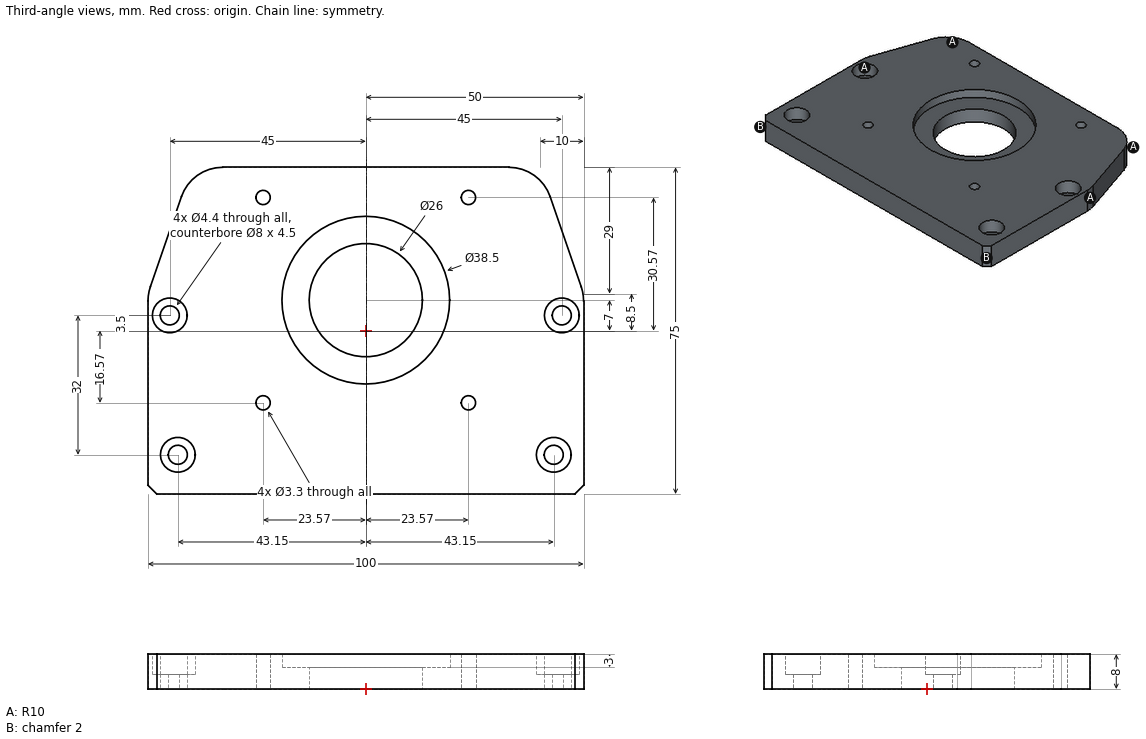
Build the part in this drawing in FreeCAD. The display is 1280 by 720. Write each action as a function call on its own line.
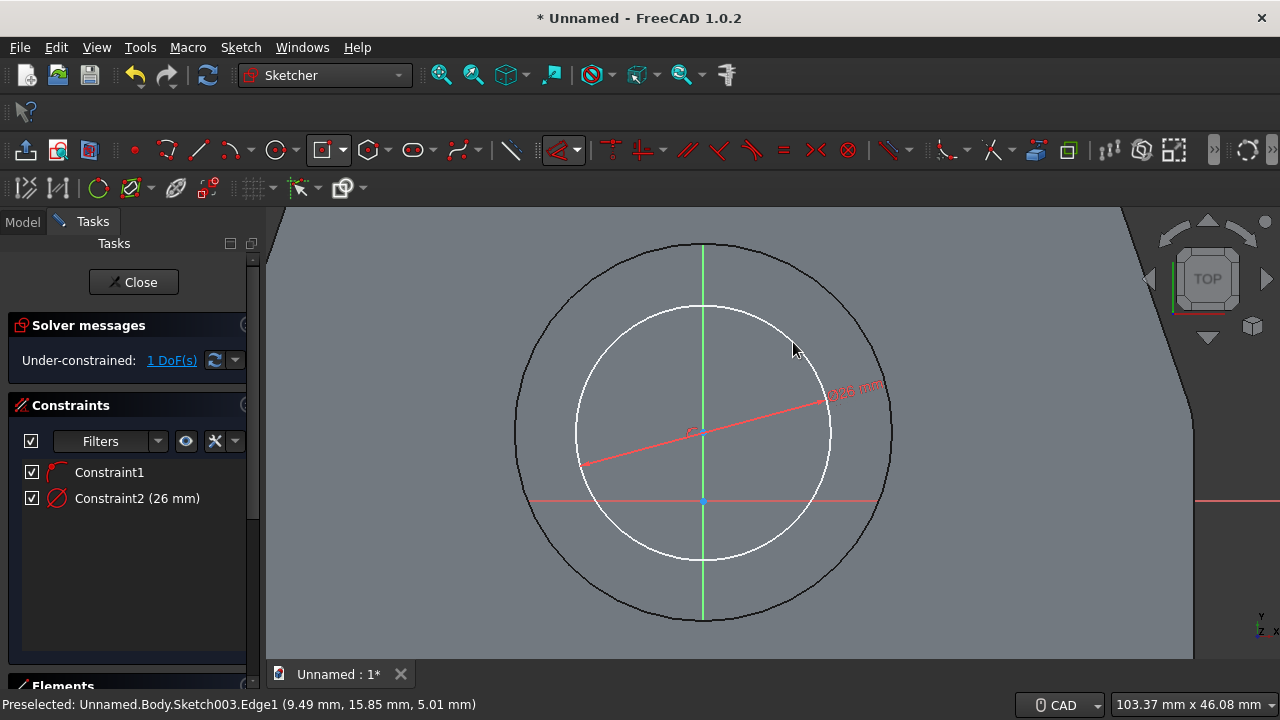
click(703, 433)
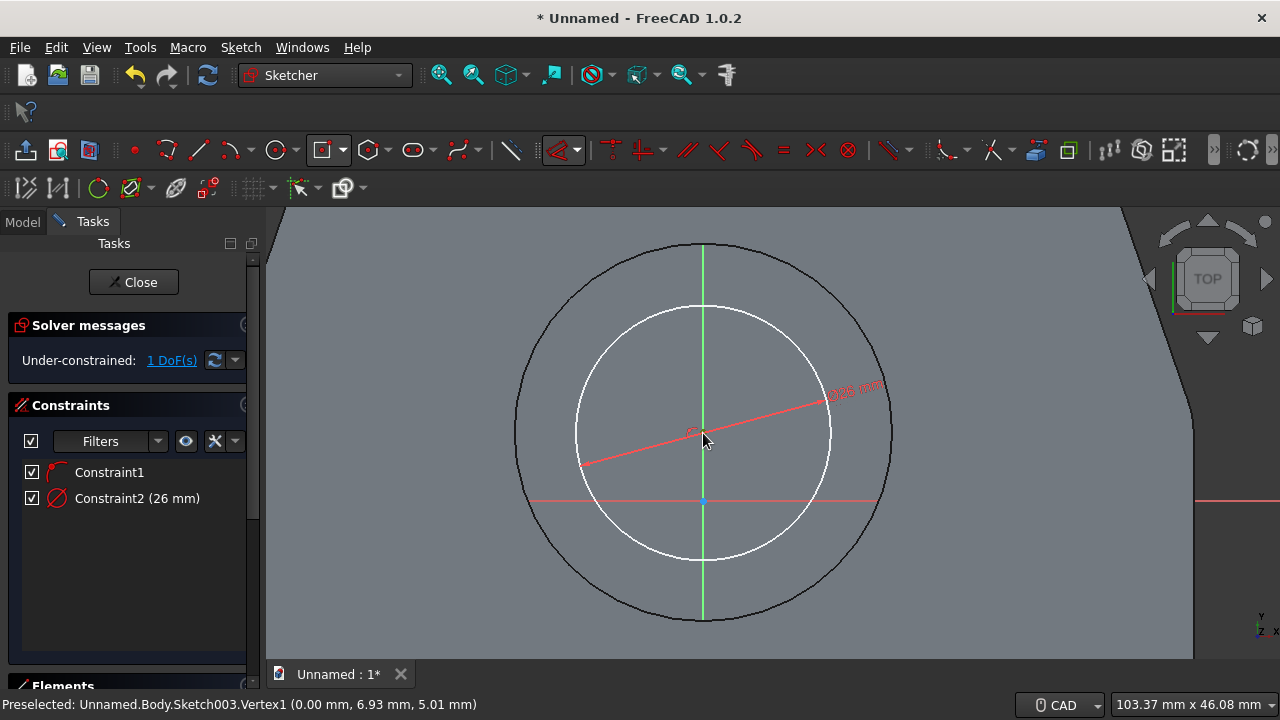
key(i)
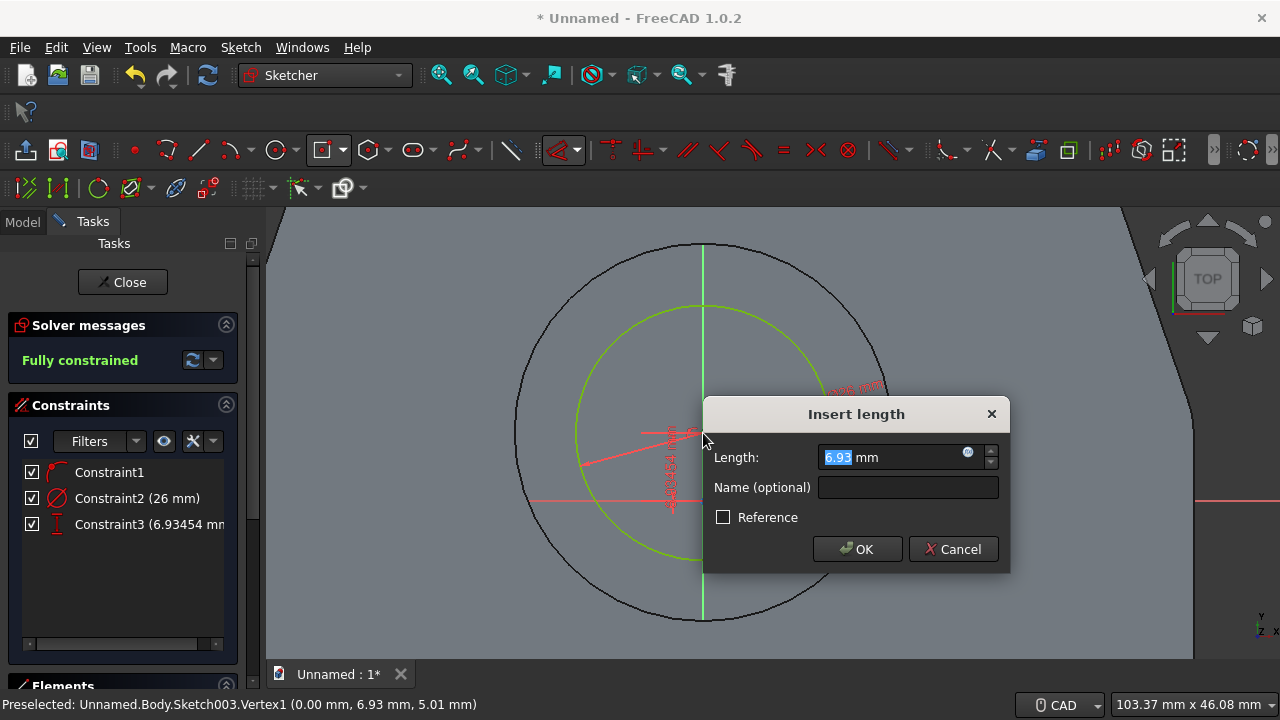
text(7)
key(Return)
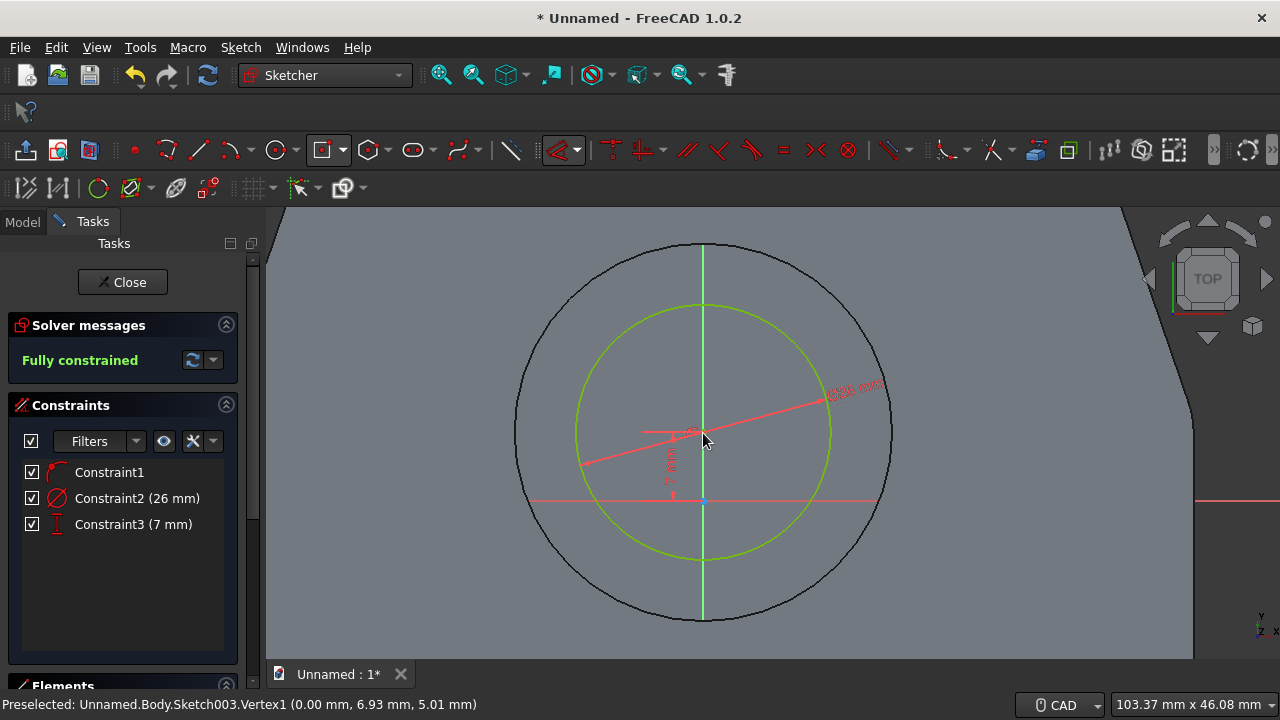
click(123, 282)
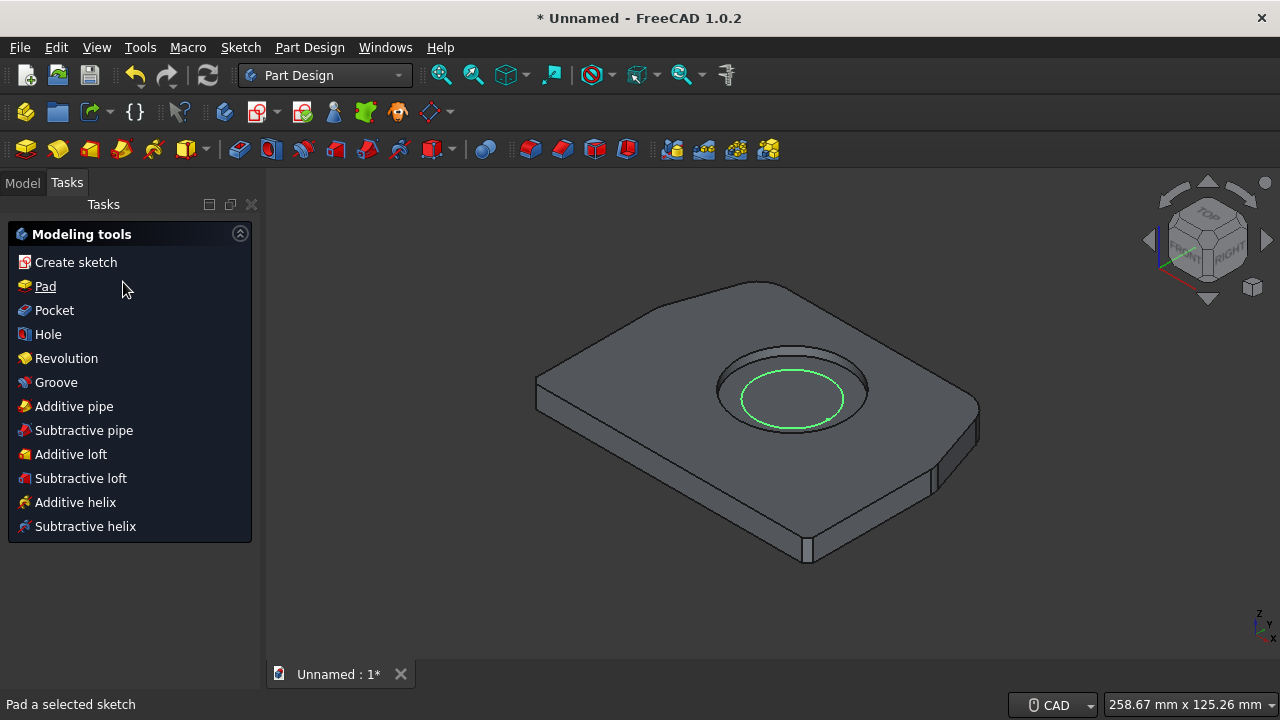
click(240, 150)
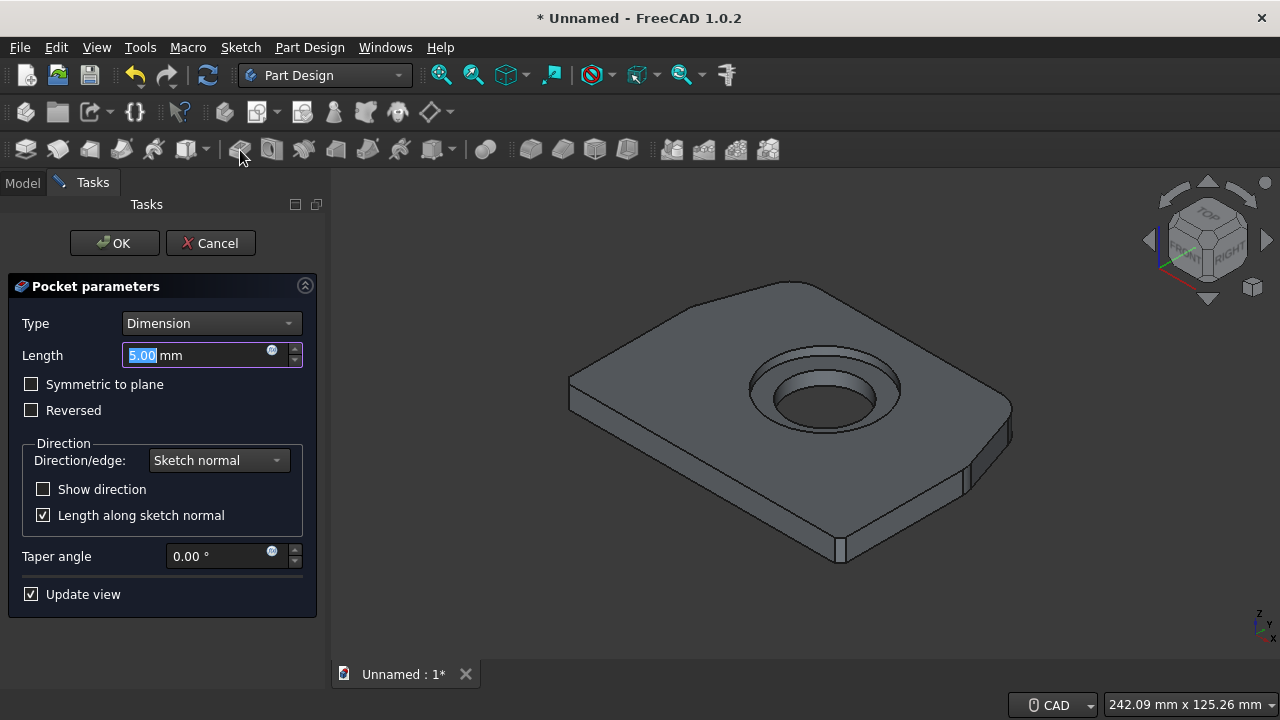
click(212, 324)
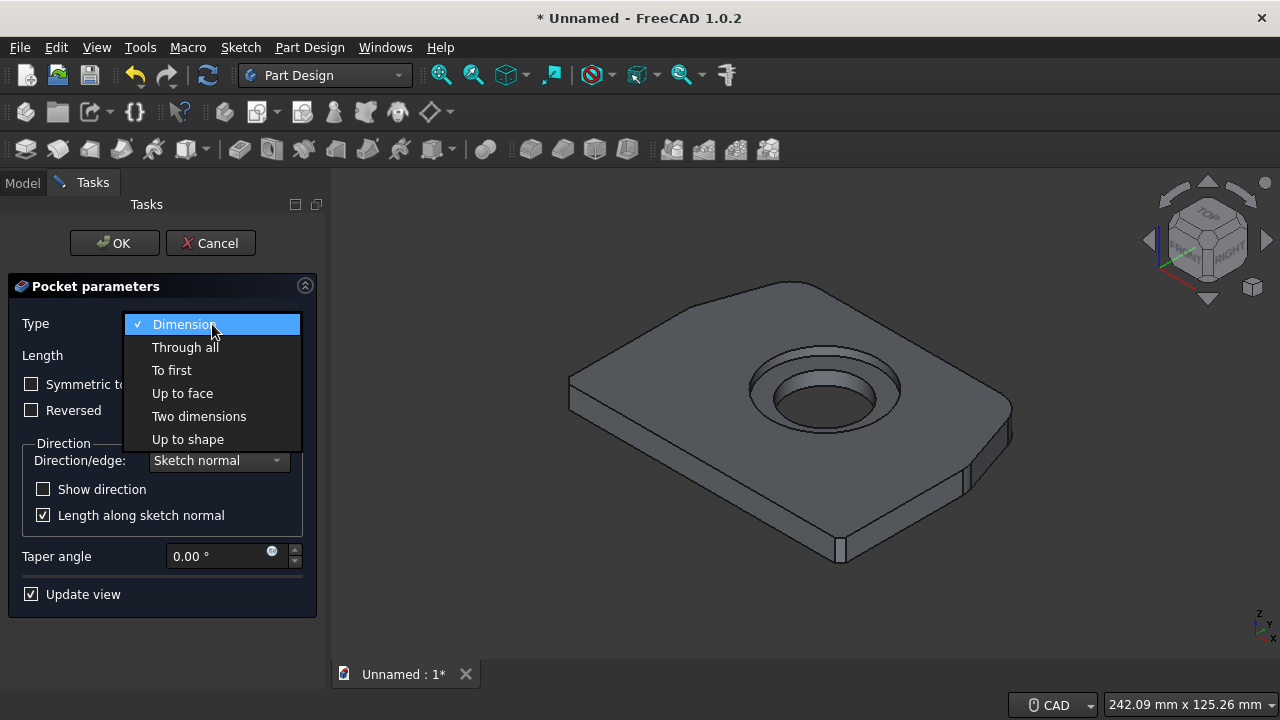
click(212, 348)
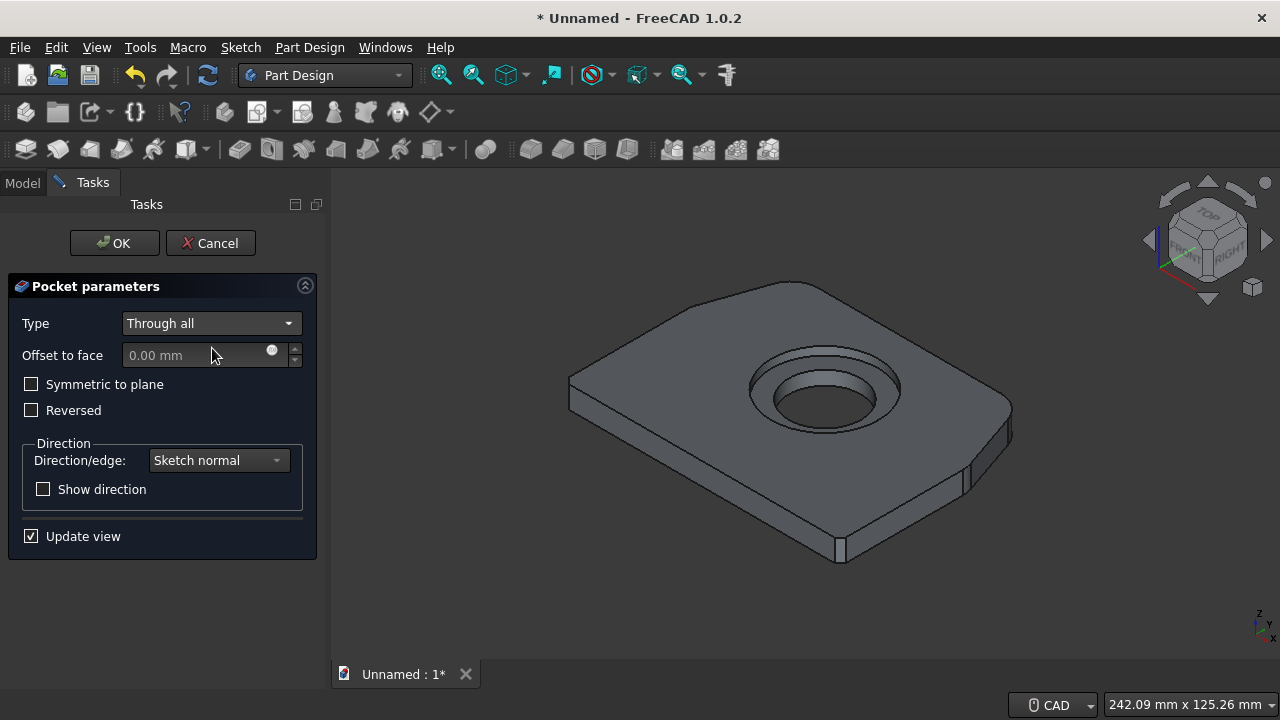
click(115, 243)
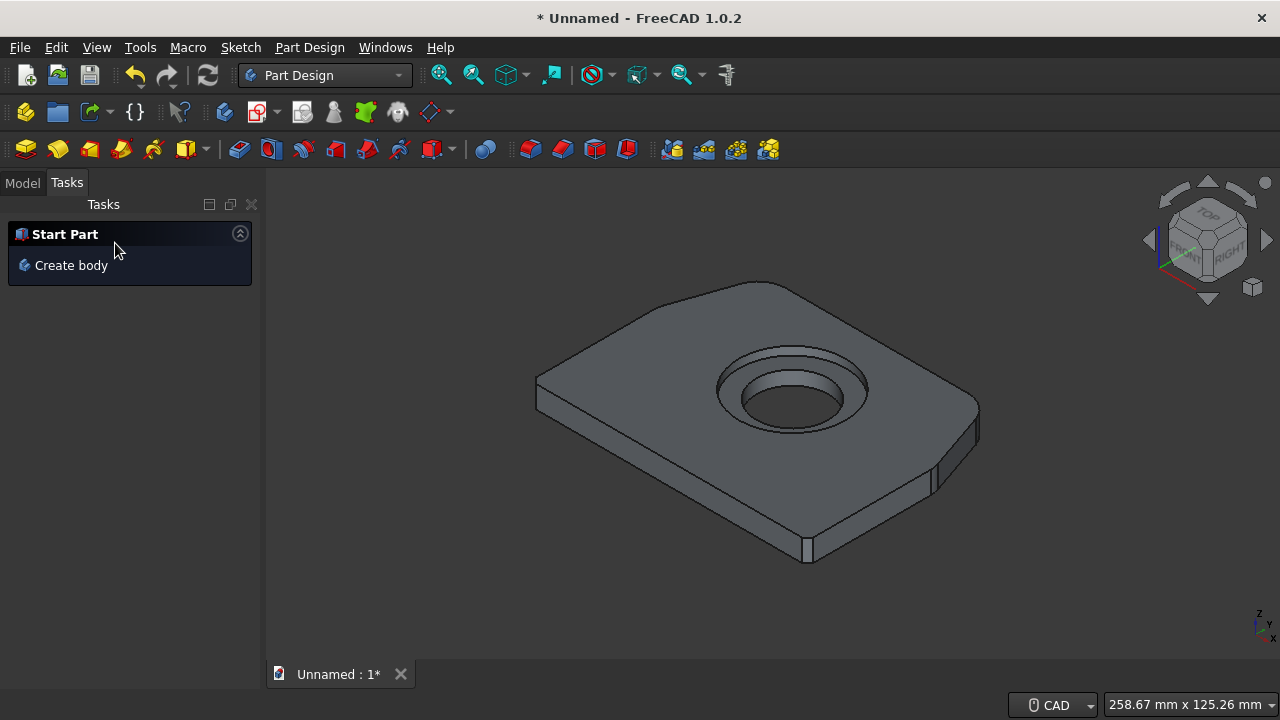
click(793, 480)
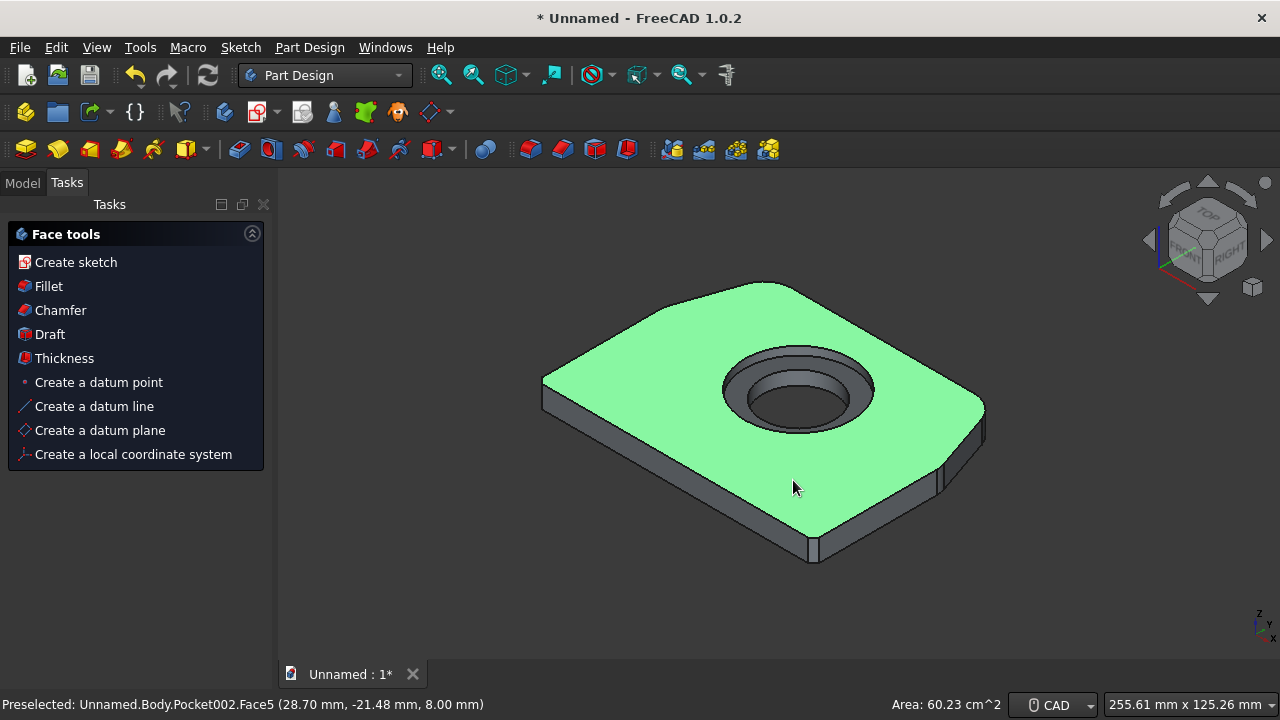
click(258, 112)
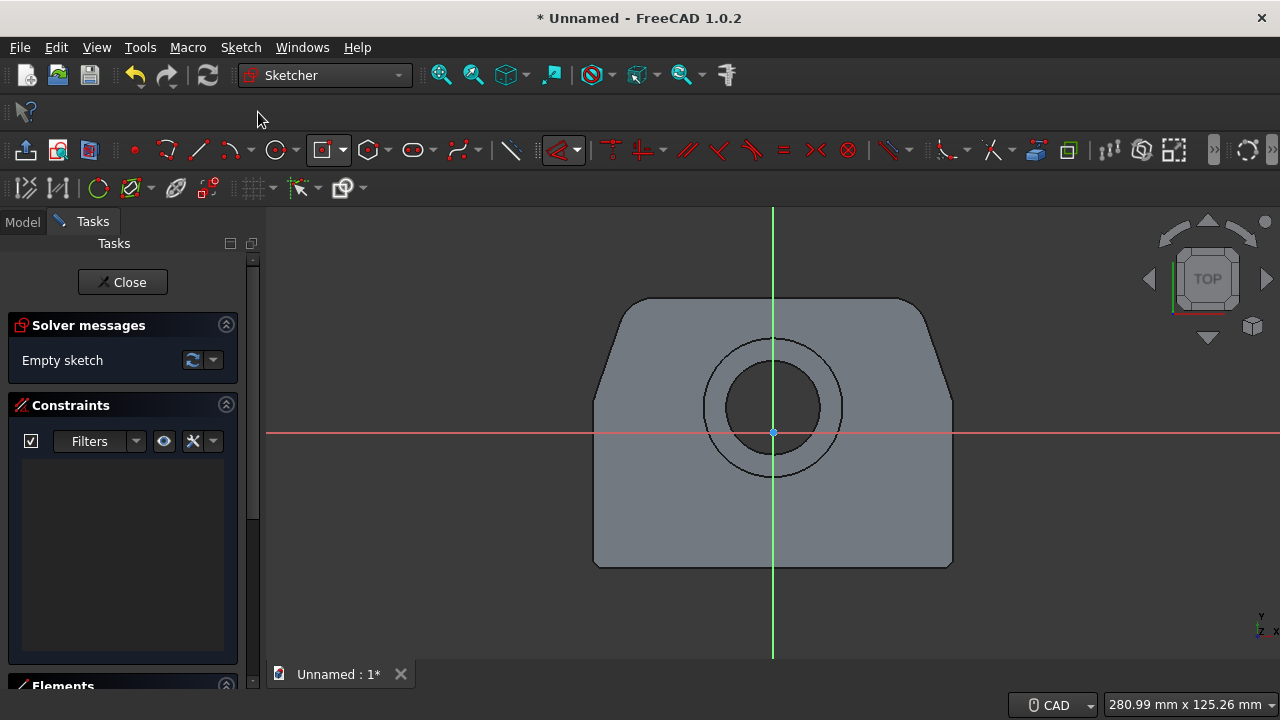
scroll(856, 533, up, 3)